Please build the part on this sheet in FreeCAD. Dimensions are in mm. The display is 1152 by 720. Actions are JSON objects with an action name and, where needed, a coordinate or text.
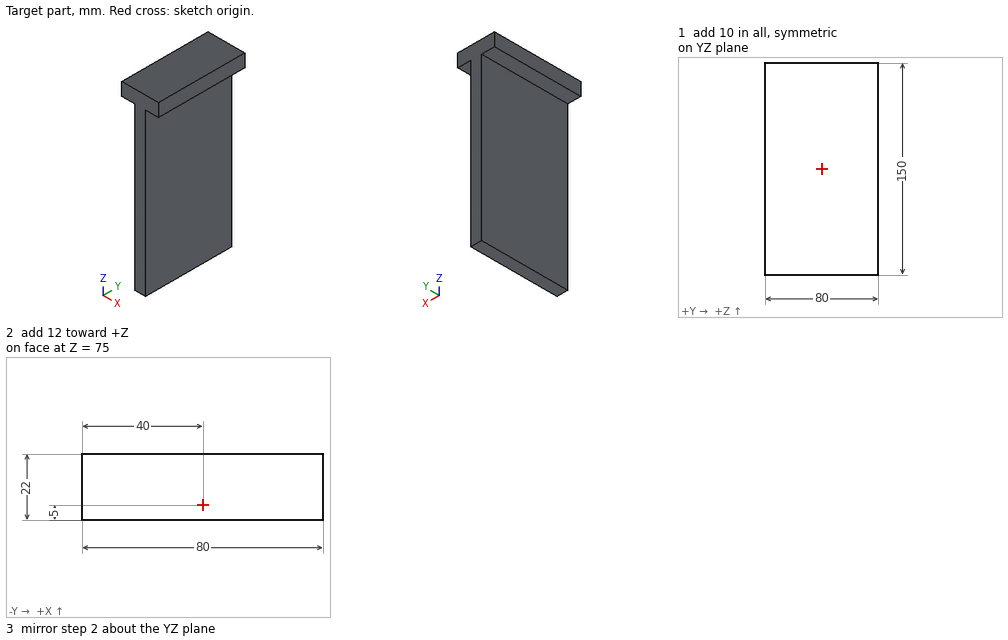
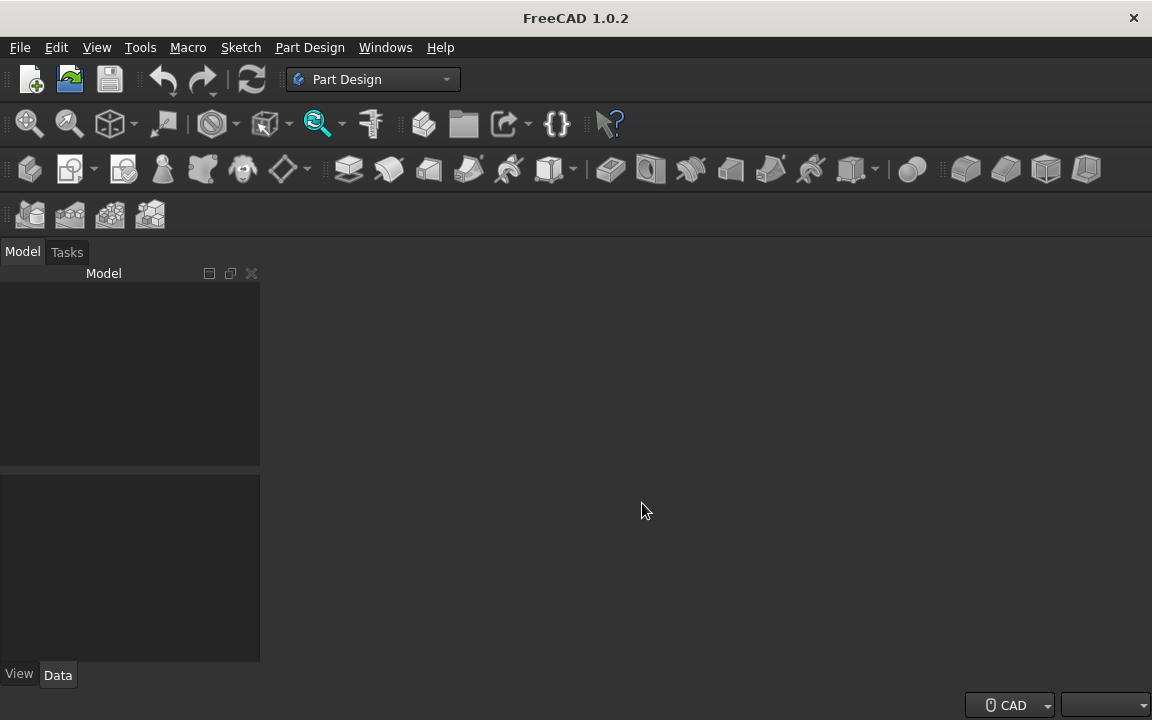
{"action": "left_click", "coordinate": [30, 80]}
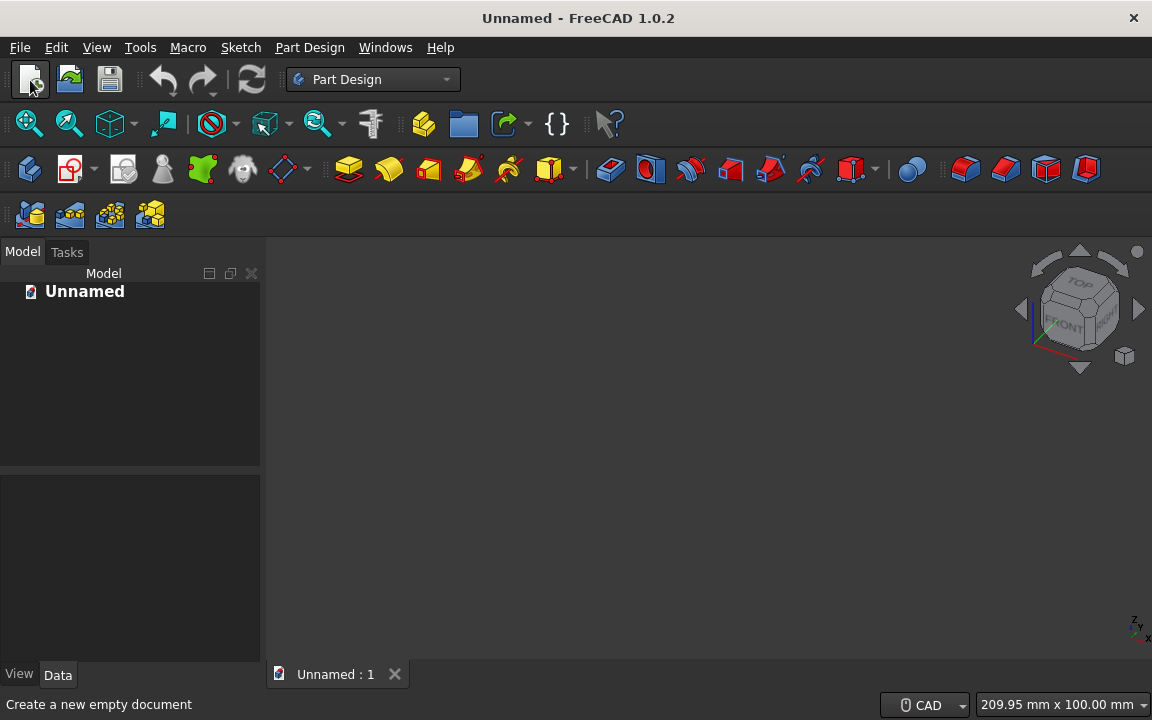
{"action": "left_click", "coordinate": [70, 170]}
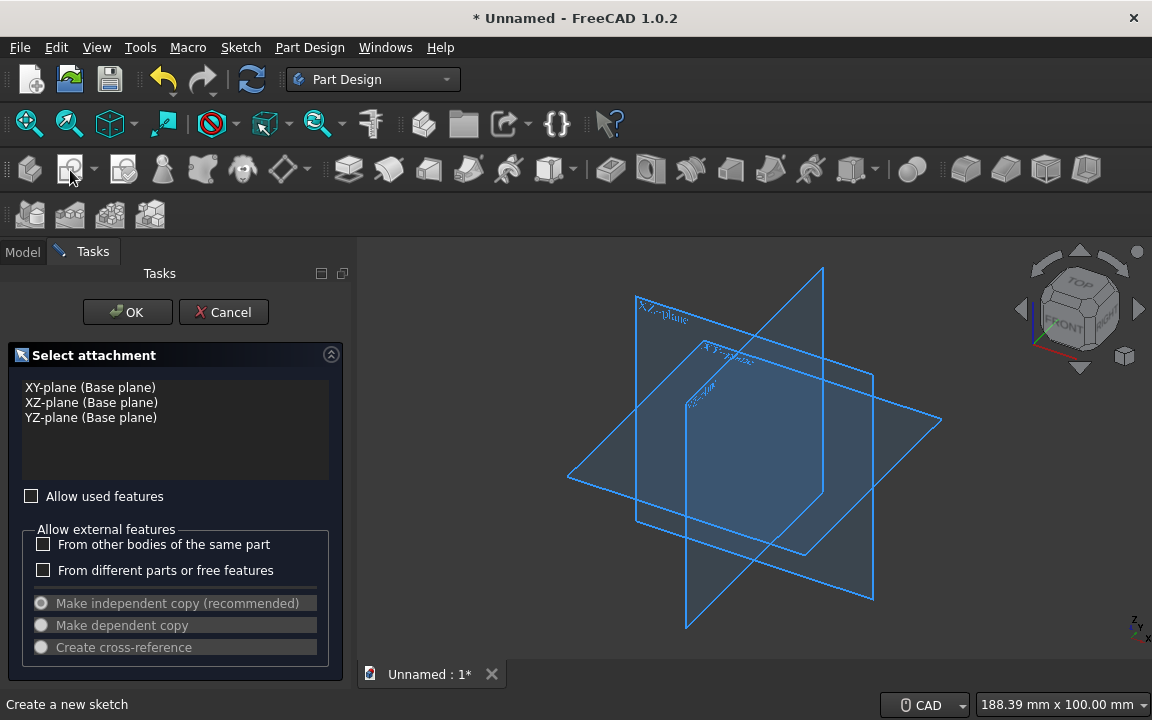
{"action": "left_click", "coordinate": [82, 418]}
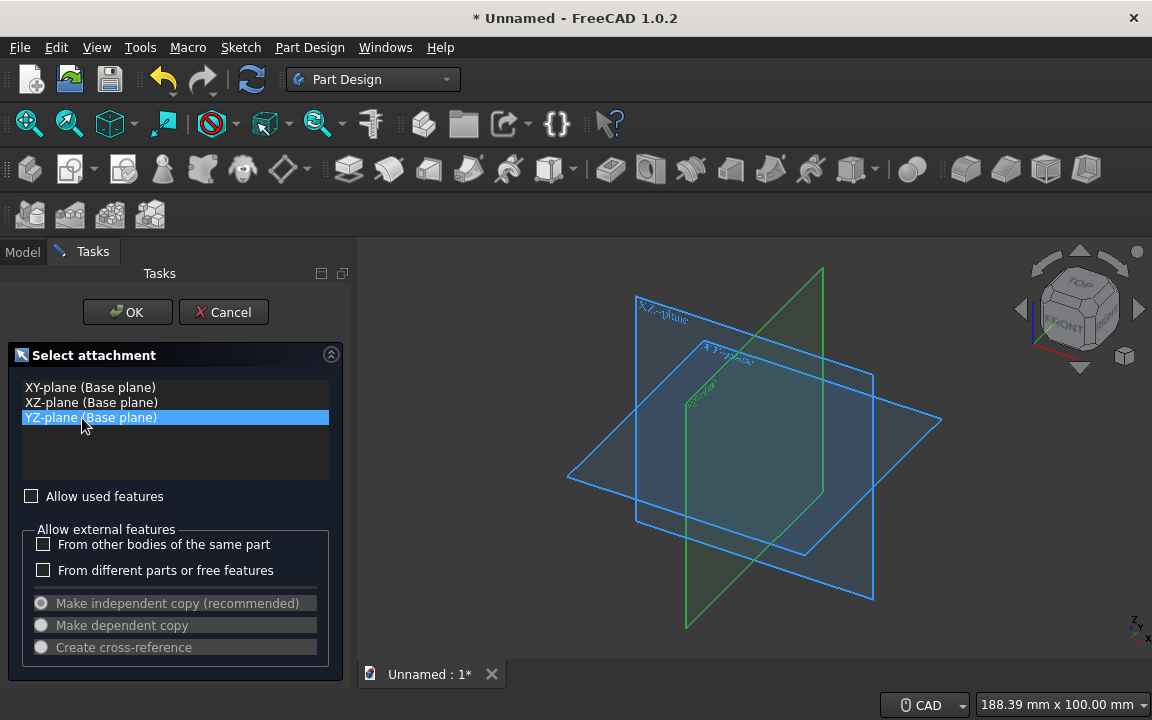
{"action": "left_click", "coordinate": [128, 312]}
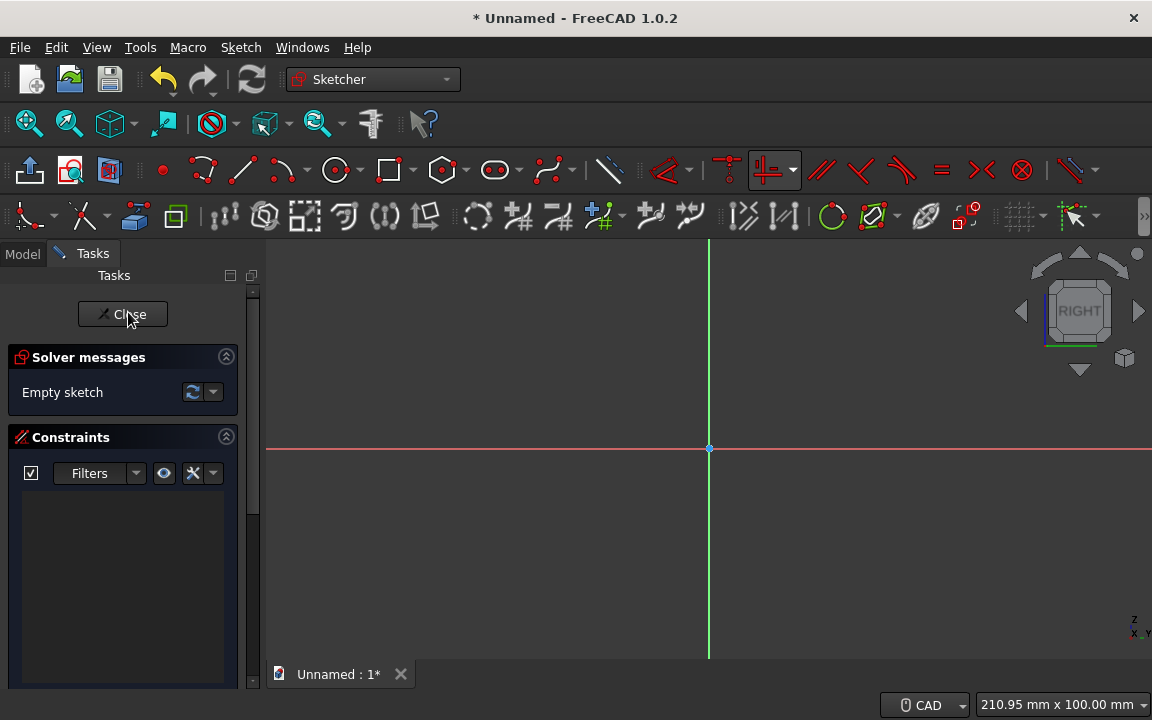
{"action": "scroll", "coordinate": [585, 449], "scroll_direction": "down", "scroll_amount": 4}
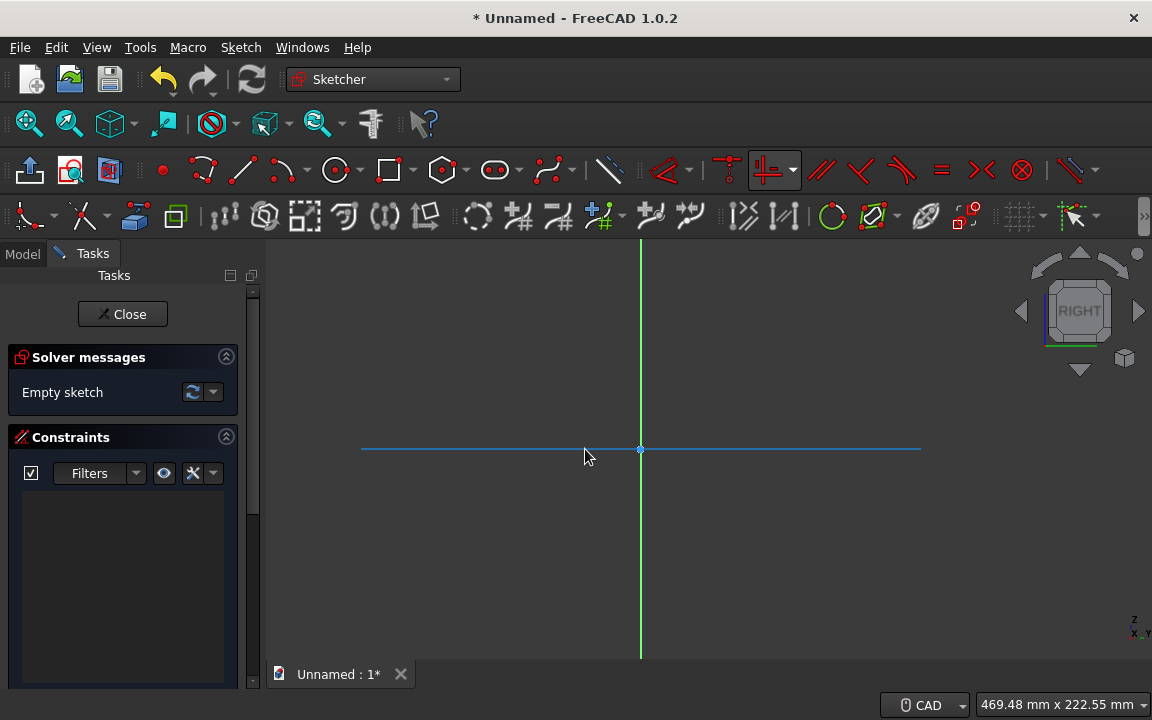
{"action": "left_click", "coordinate": [416, 170]}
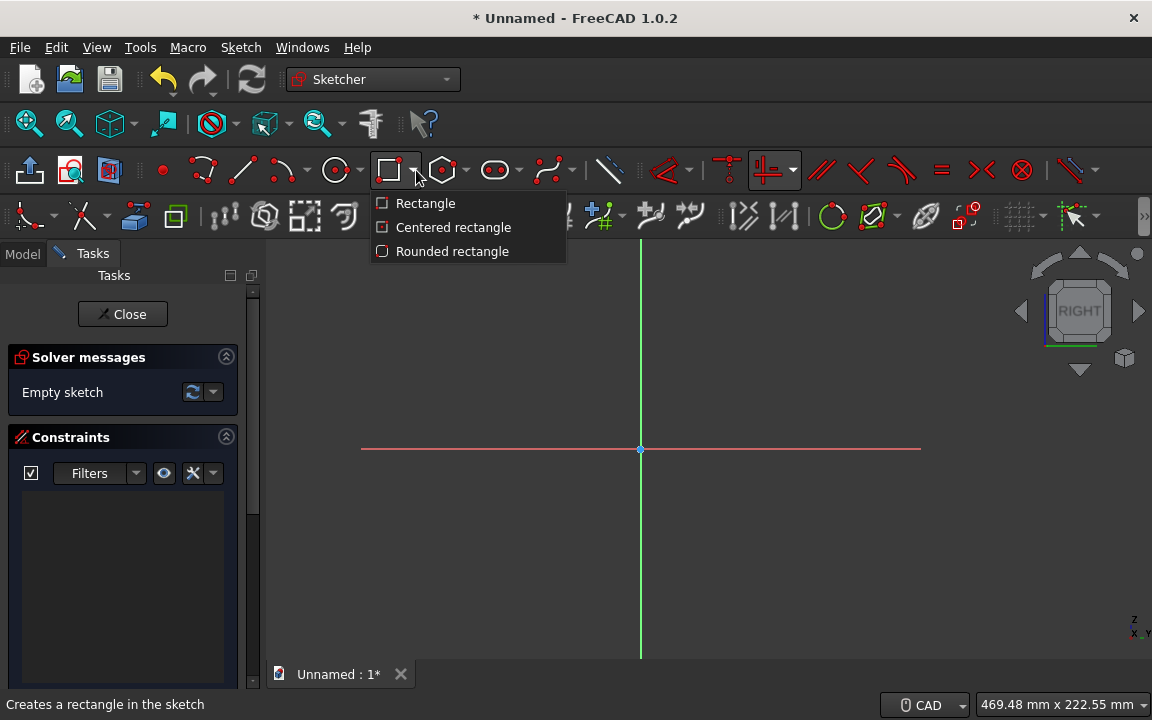
{"action": "left_click", "coordinate": [468, 227]}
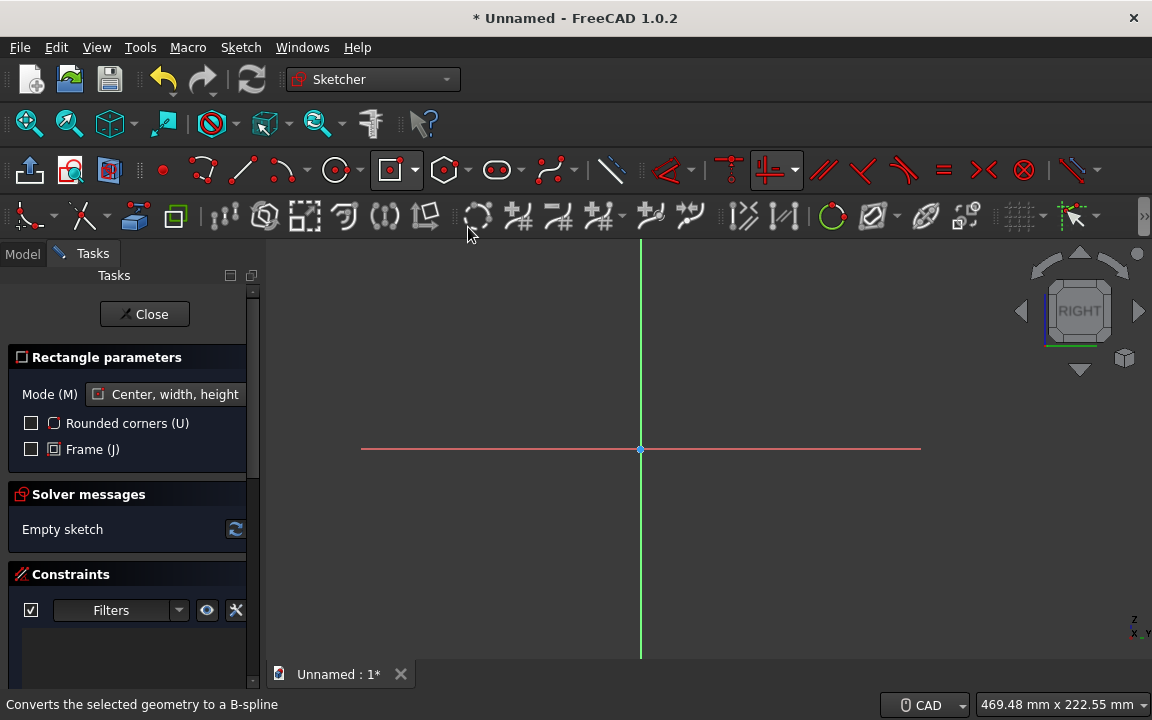
{"action": "left_click", "coordinate": [641, 449]}
{"action": "left_click", "coordinate": [716, 308]}
{"action": "key", "text": "Escape"}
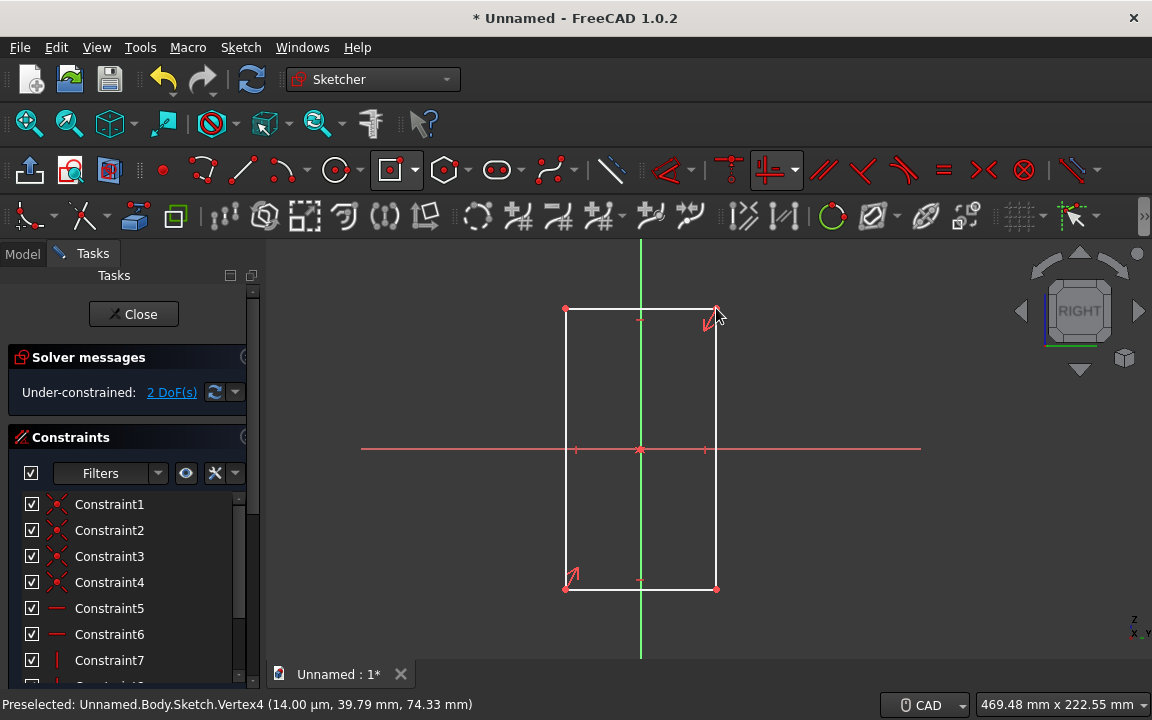
{"action": "left_click", "coordinate": [666, 170]}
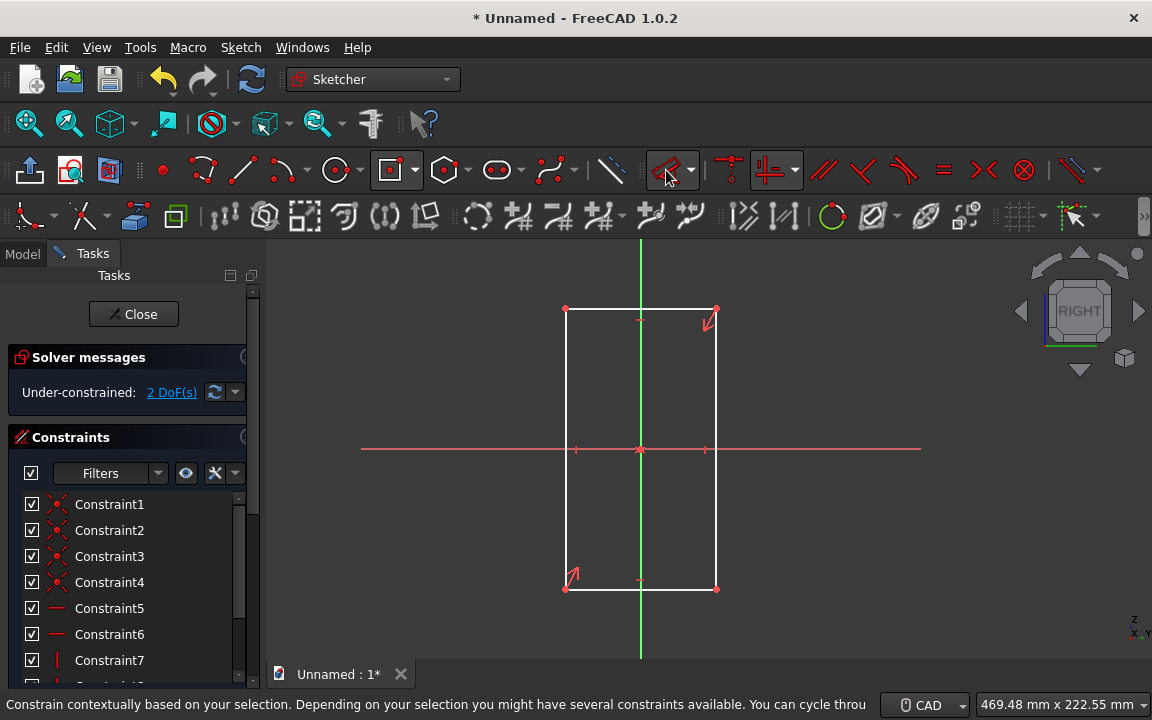
{"action": "left_click", "coordinate": [611, 590]}
{"action": "left_click", "coordinate": [606, 624]}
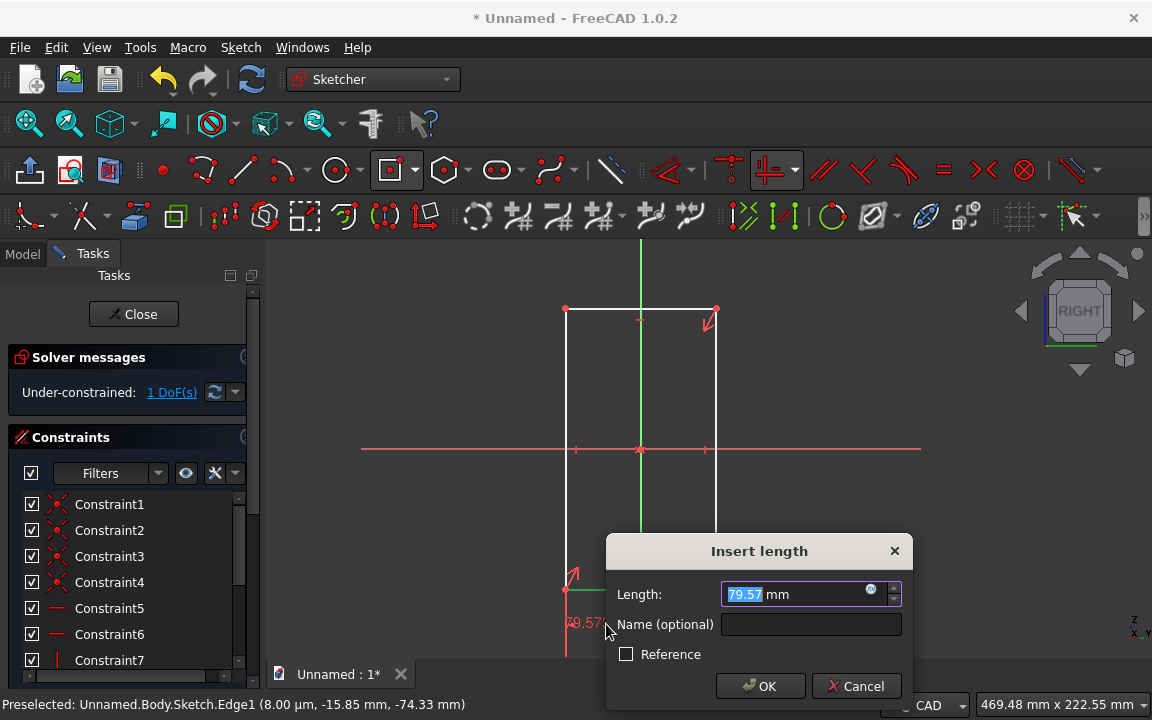
{"action": "type", "text": "80"}
{"action": "key", "text": "Return"}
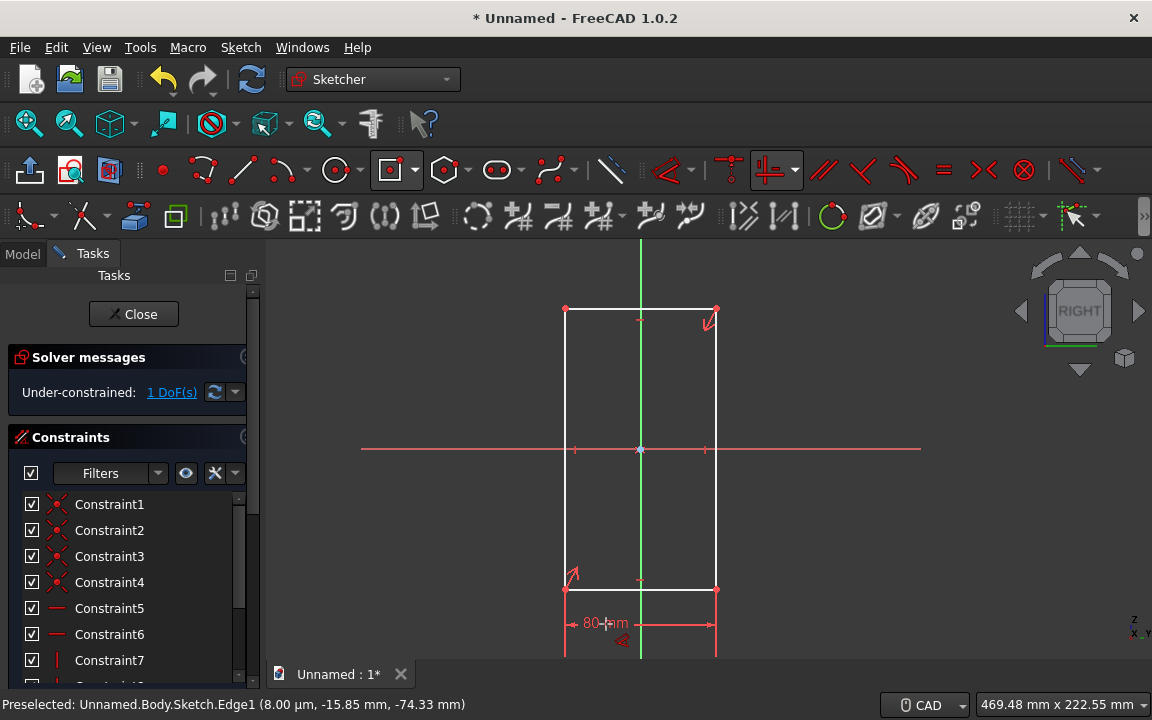
{"action": "left_click", "coordinate": [716, 505]}
{"action": "left_click", "coordinate": [750, 385]}